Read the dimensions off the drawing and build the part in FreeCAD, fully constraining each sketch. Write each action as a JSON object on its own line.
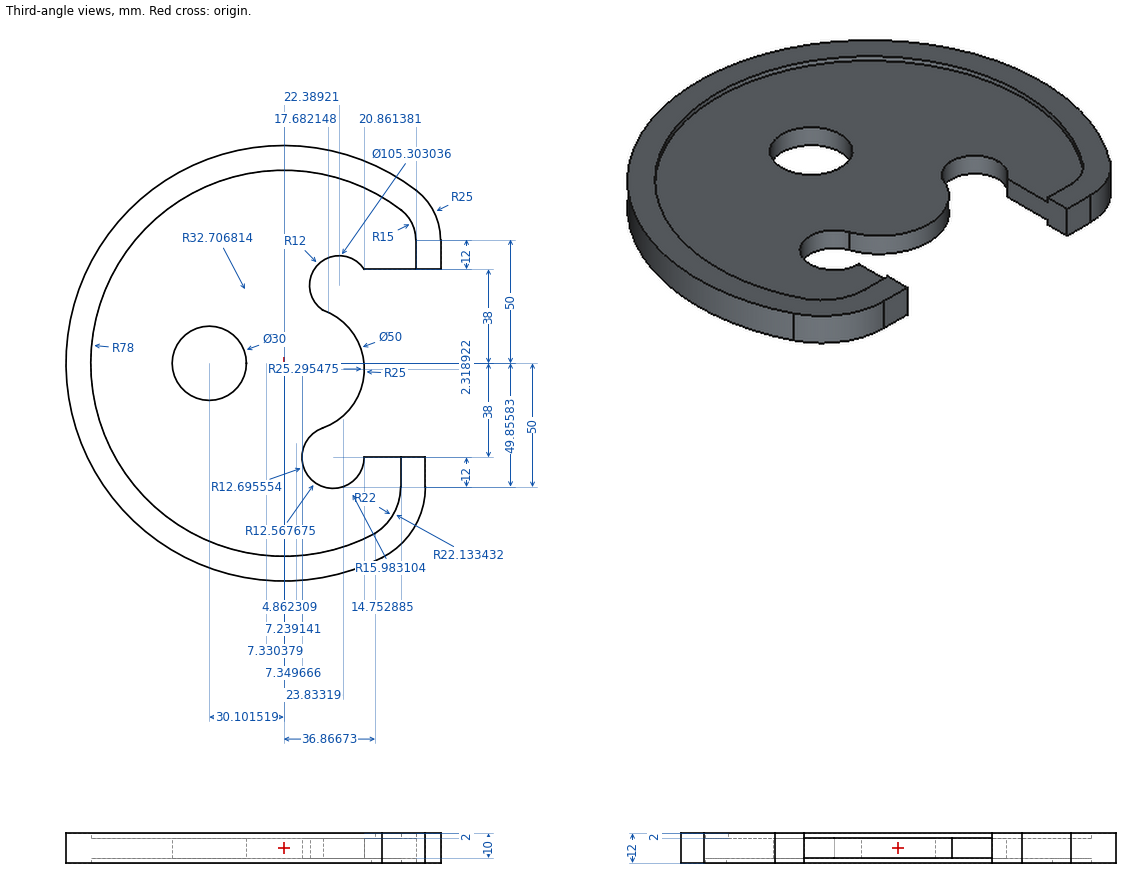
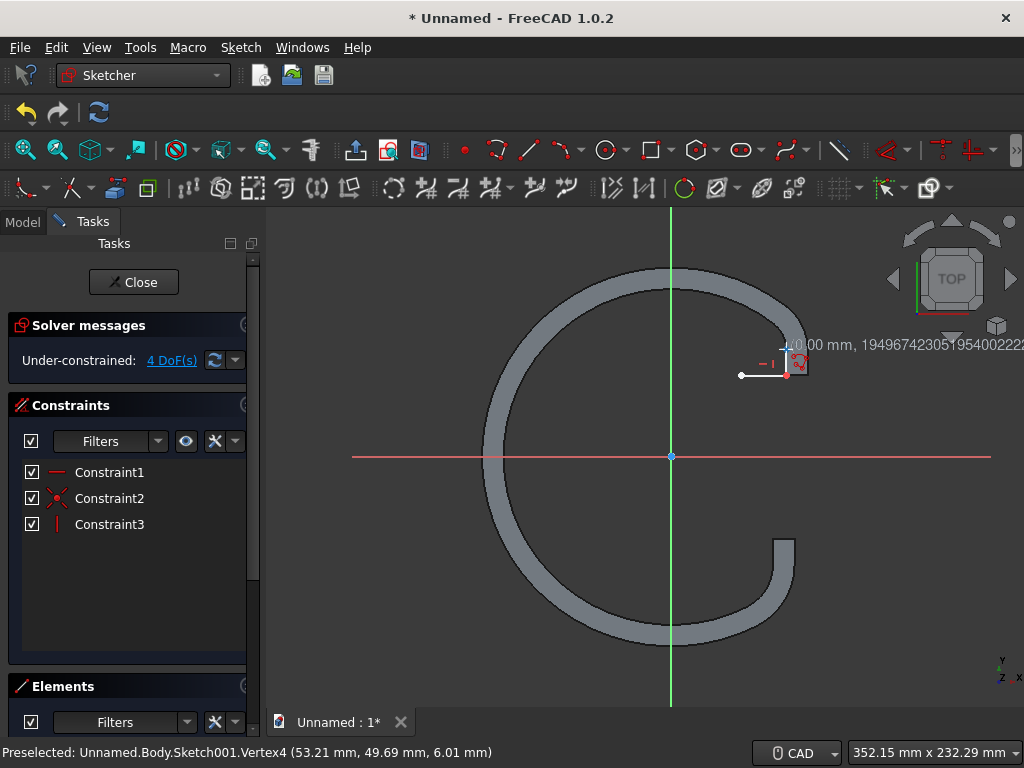
{"action": "left_click", "coordinate": [773, 565]}
{"action": "left_click", "coordinate": [773, 539]}
{"action": "left_click", "coordinate": [741, 539]}
{"action": "right_click", "coordinate": [741, 539]}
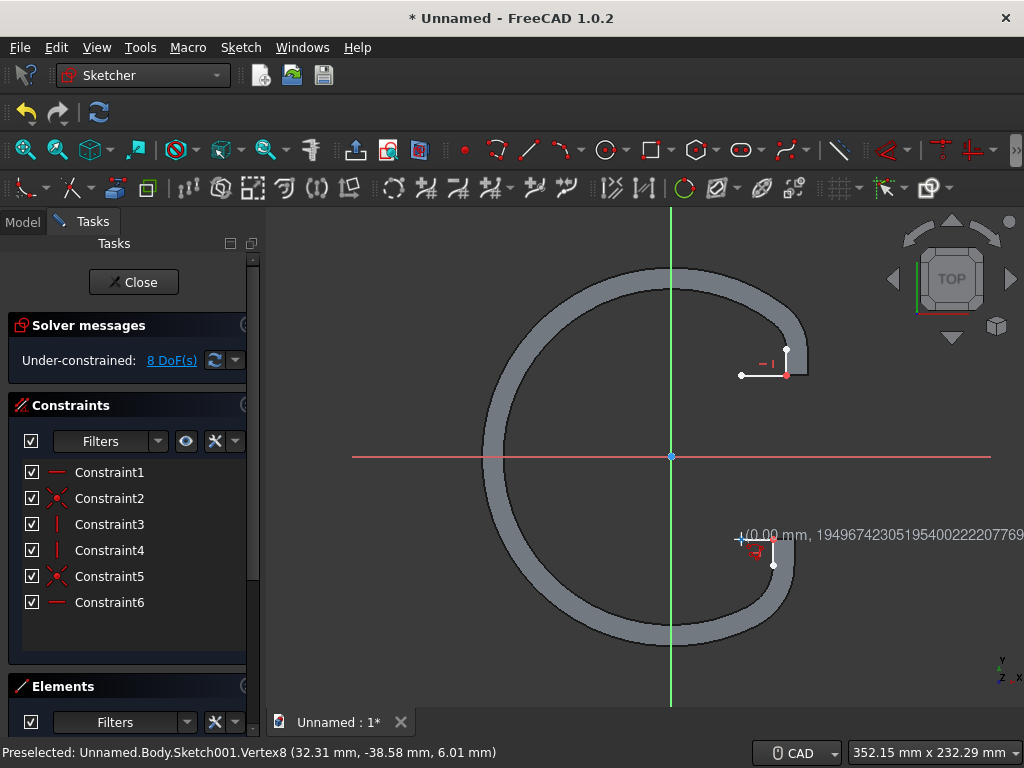
{"action": "left_click", "coordinate": [562, 150]}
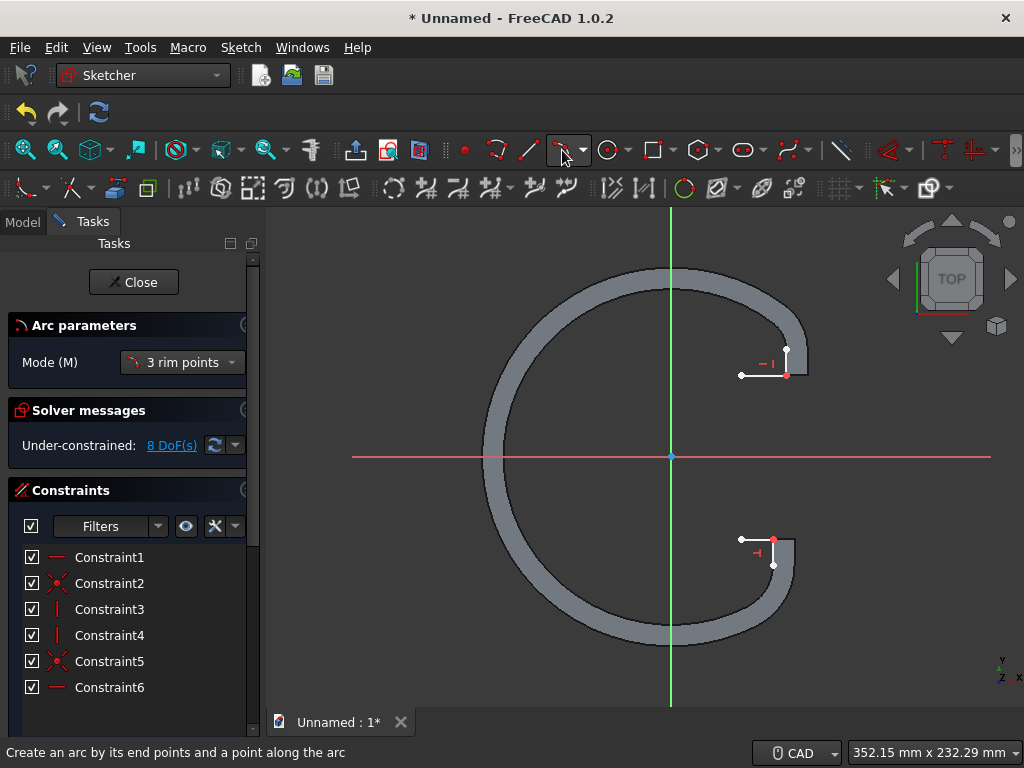
{"action": "scroll", "coordinate": [786, 349], "scroll_direction": "up", "scroll_amount": 2}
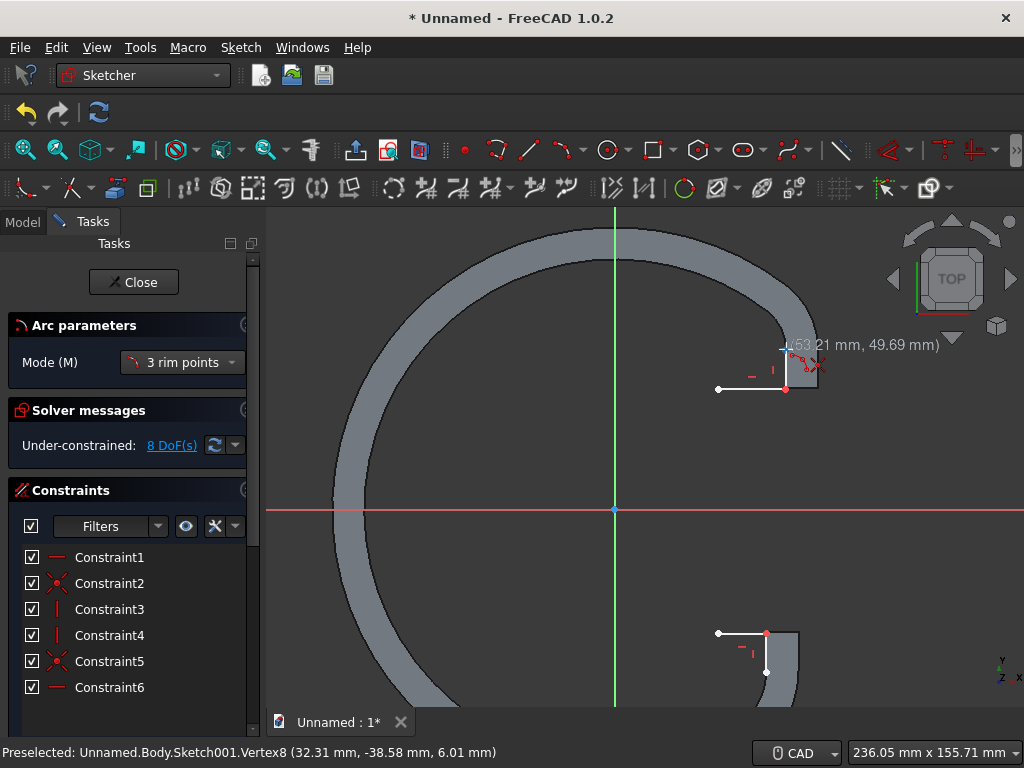
{"action": "left_click", "coordinate": [786, 350]}
{"action": "left_click", "coordinate": [767, 311]}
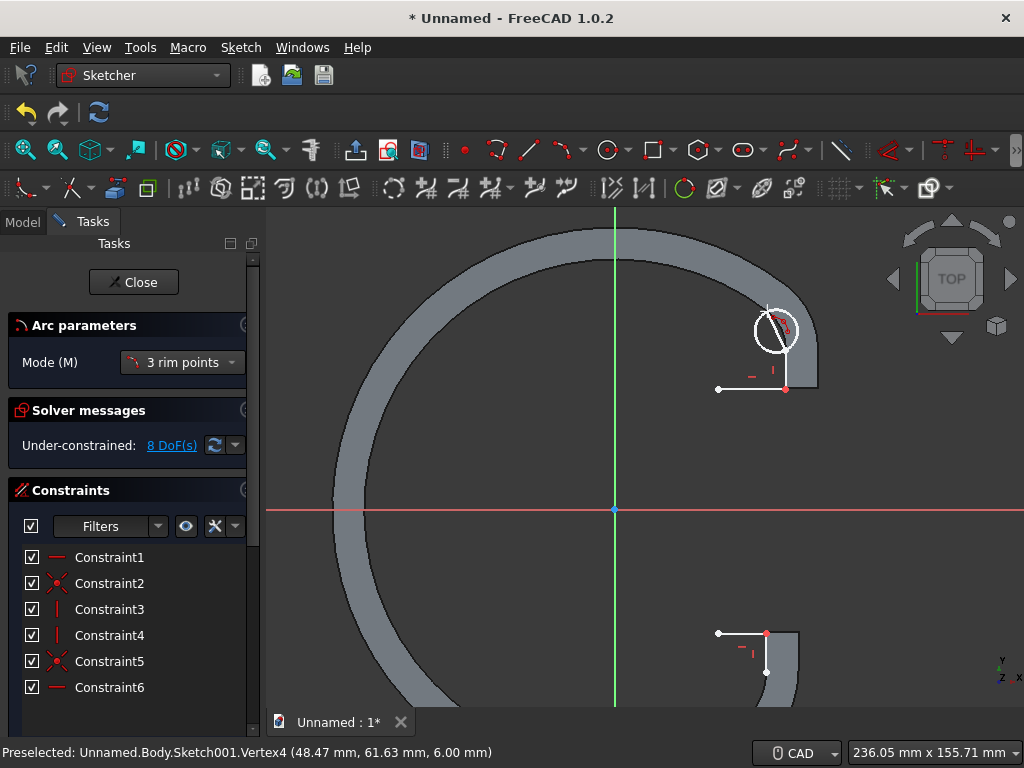
{"action": "scroll", "coordinate": [781, 328], "scroll_direction": "up", "scroll_amount": 6}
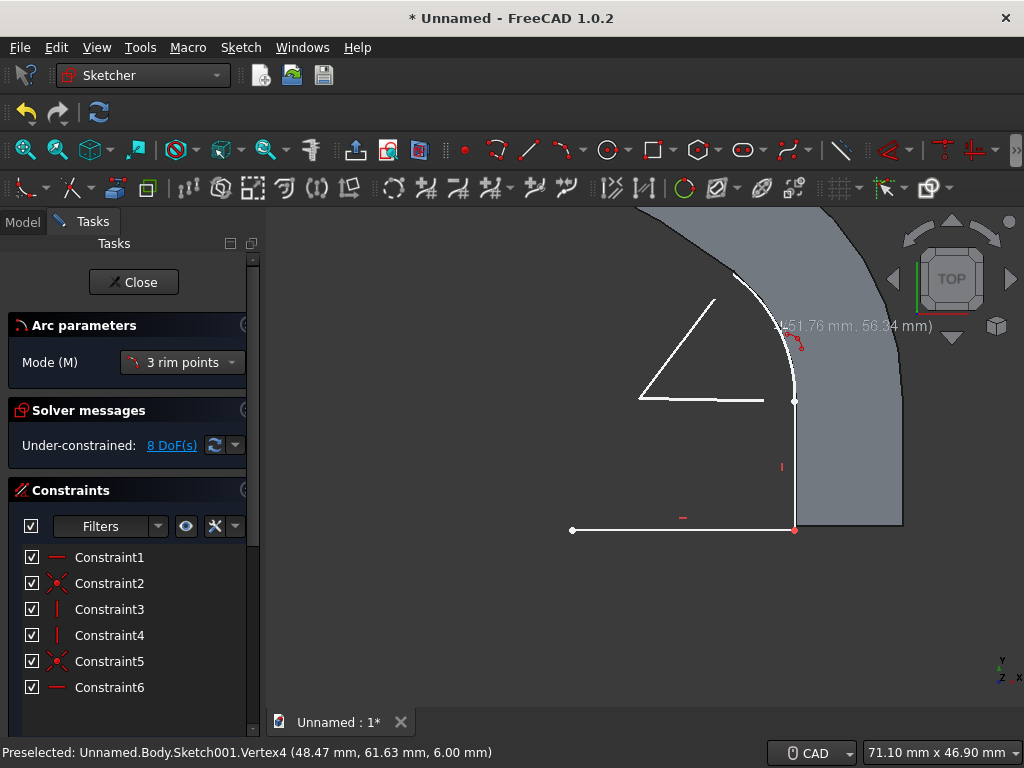
{"action": "left_click", "coordinate": [780, 328]}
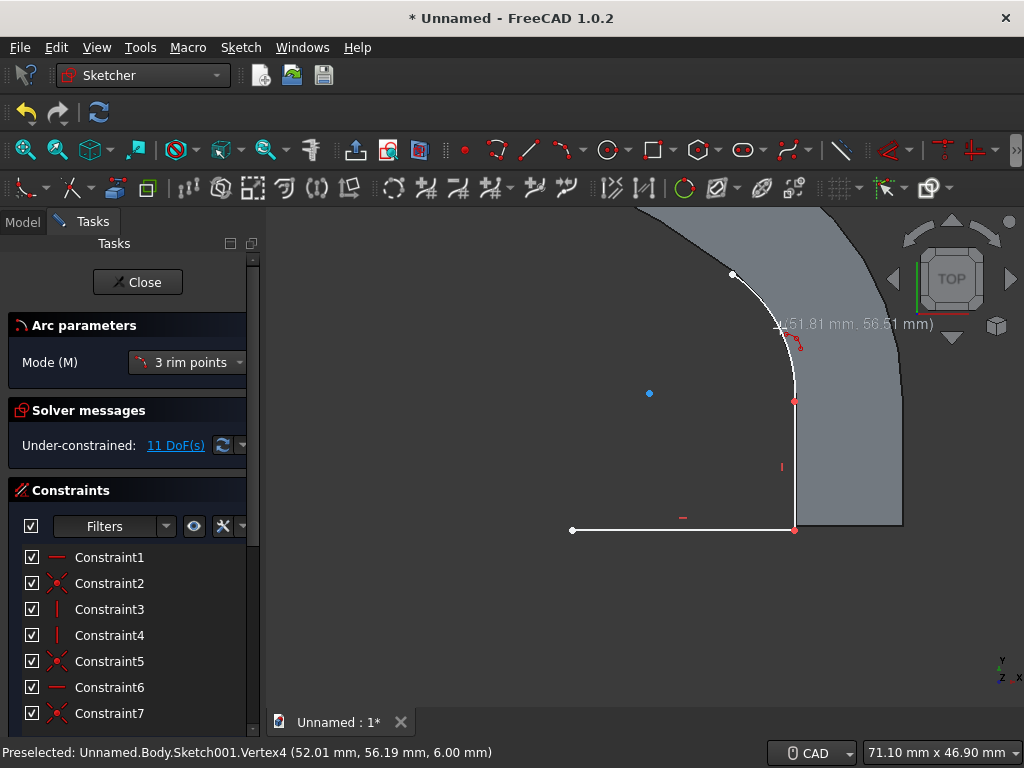
{"action": "scroll", "coordinate": [733, 288], "scroll_direction": "down", "scroll_amount": 7}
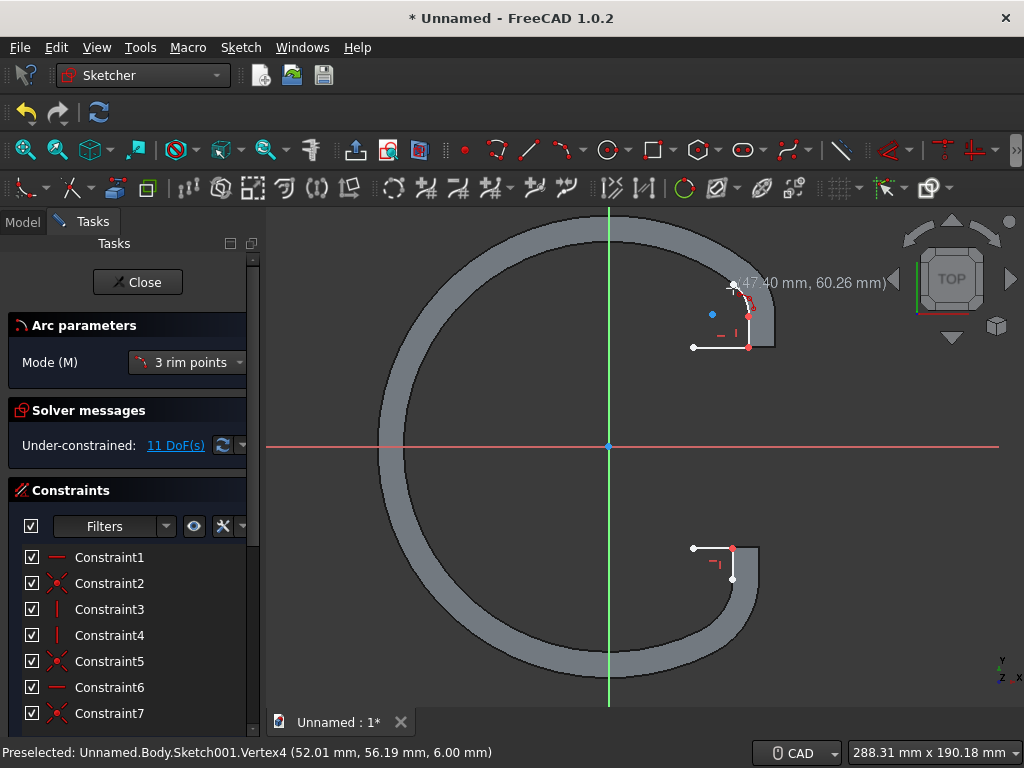
{"action": "left_click", "coordinate": [733, 285]}
{"action": "left_click", "coordinate": [701, 630]}
{"action": "left_click", "coordinate": [405, 428]}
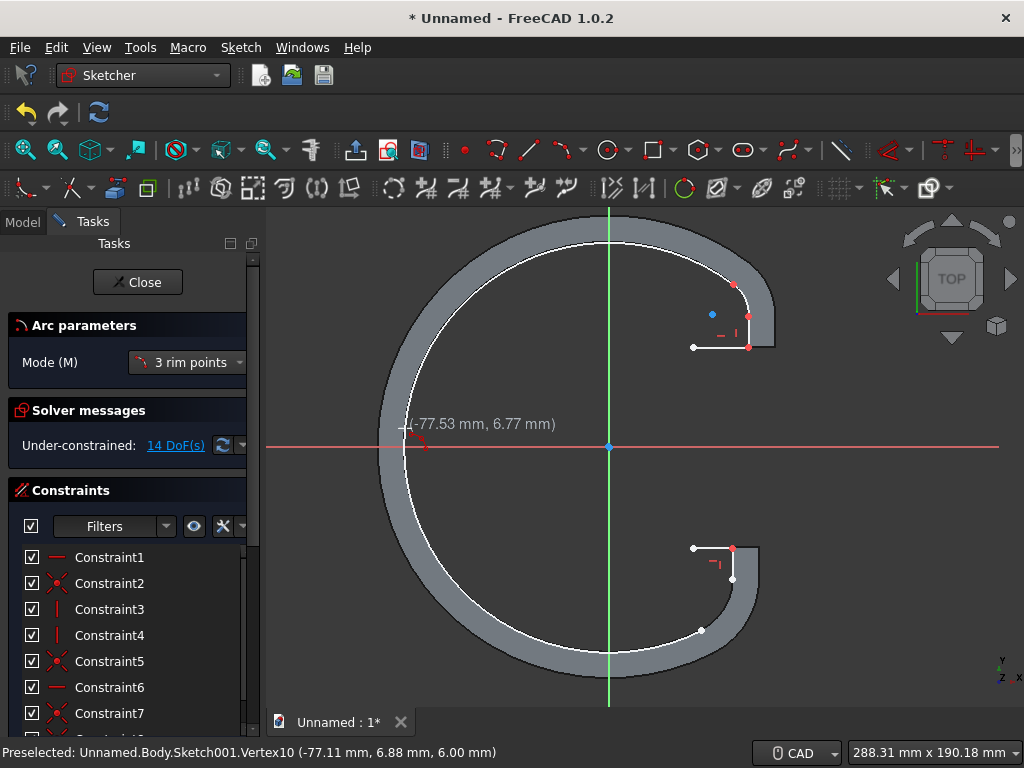
{"action": "left_click", "coordinate": [701, 631]}
{"action": "left_click", "coordinate": [733, 580]}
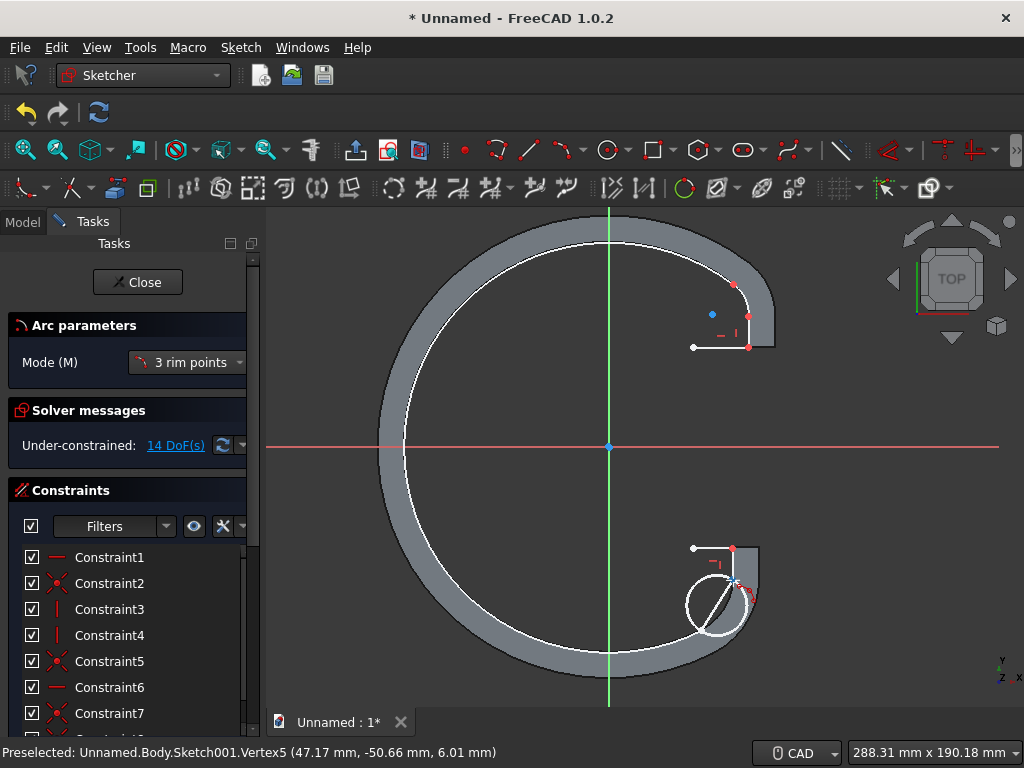
{"action": "scroll", "coordinate": [724, 609], "scroll_direction": "up", "scroll_amount": 4}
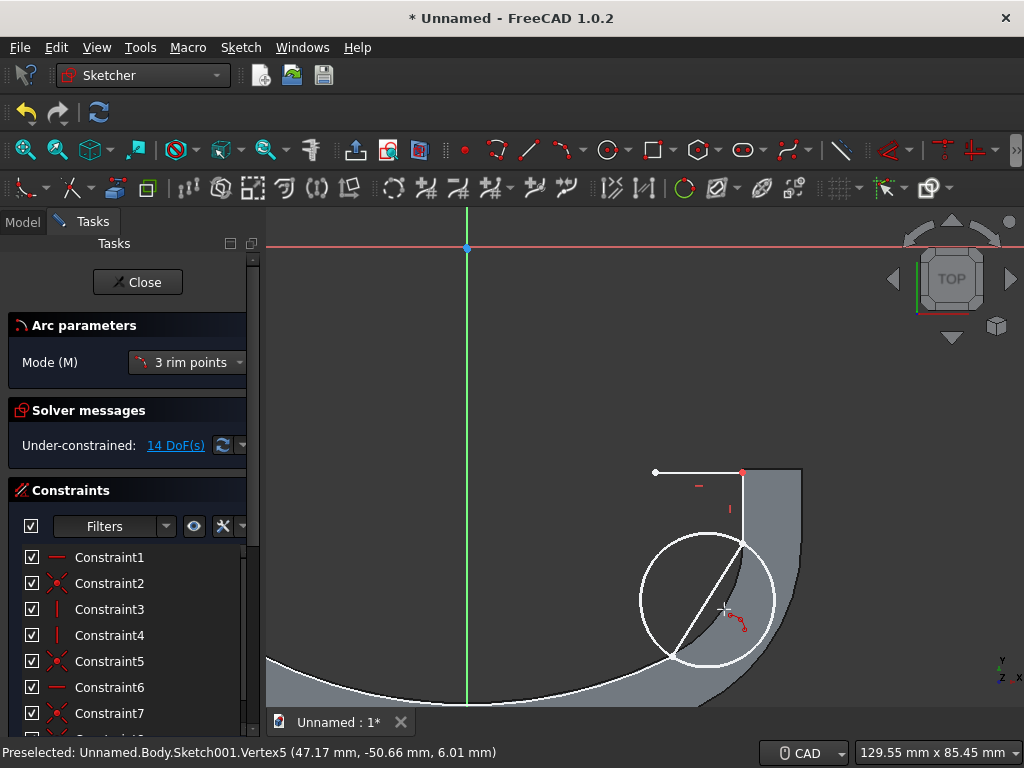
{"action": "left_click", "coordinate": [724, 607]}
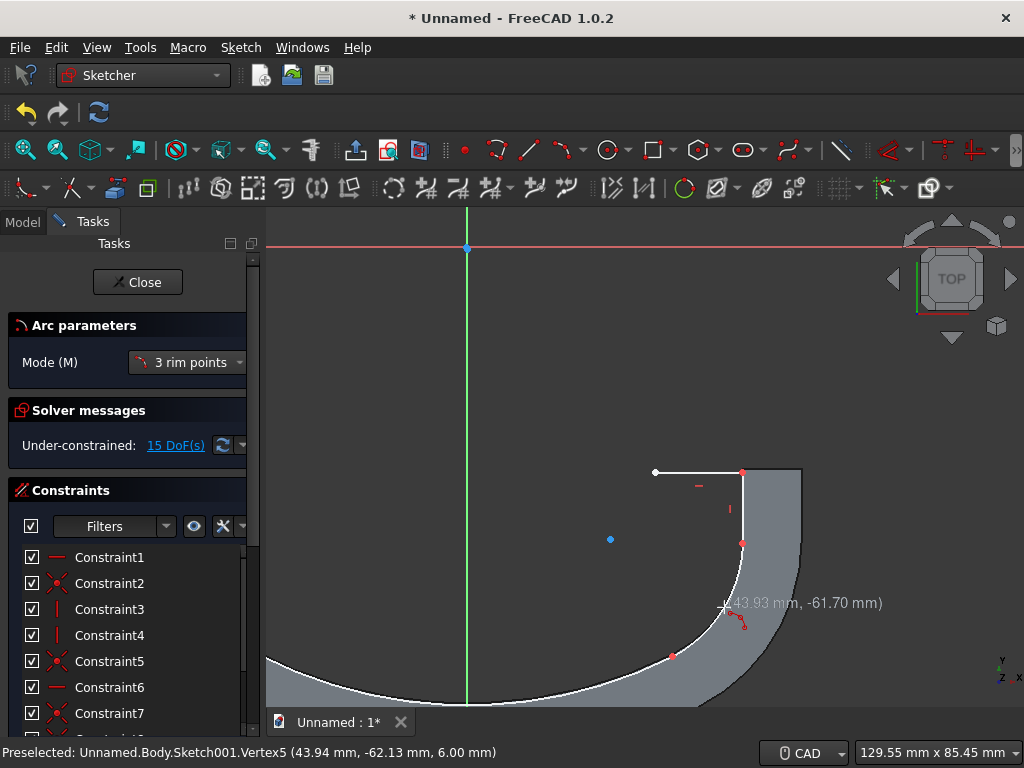
{"action": "left_click", "coordinate": [656, 473]}
{"action": "left_click", "coordinate": [559, 400]}
{"action": "left_click", "coordinate": [541, 529]}